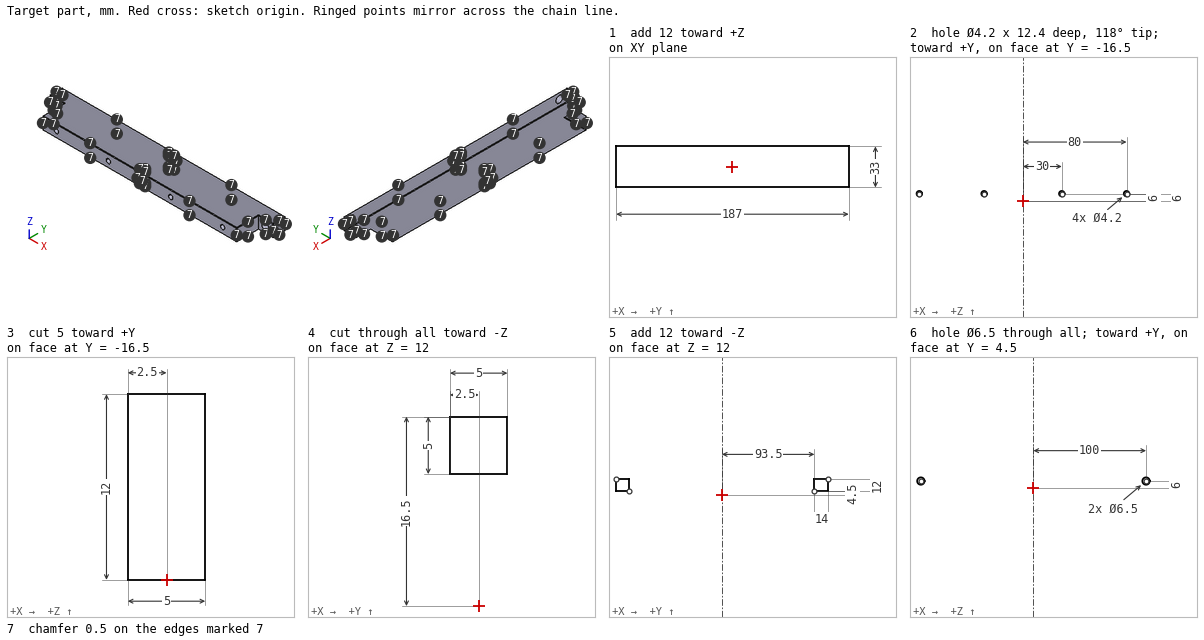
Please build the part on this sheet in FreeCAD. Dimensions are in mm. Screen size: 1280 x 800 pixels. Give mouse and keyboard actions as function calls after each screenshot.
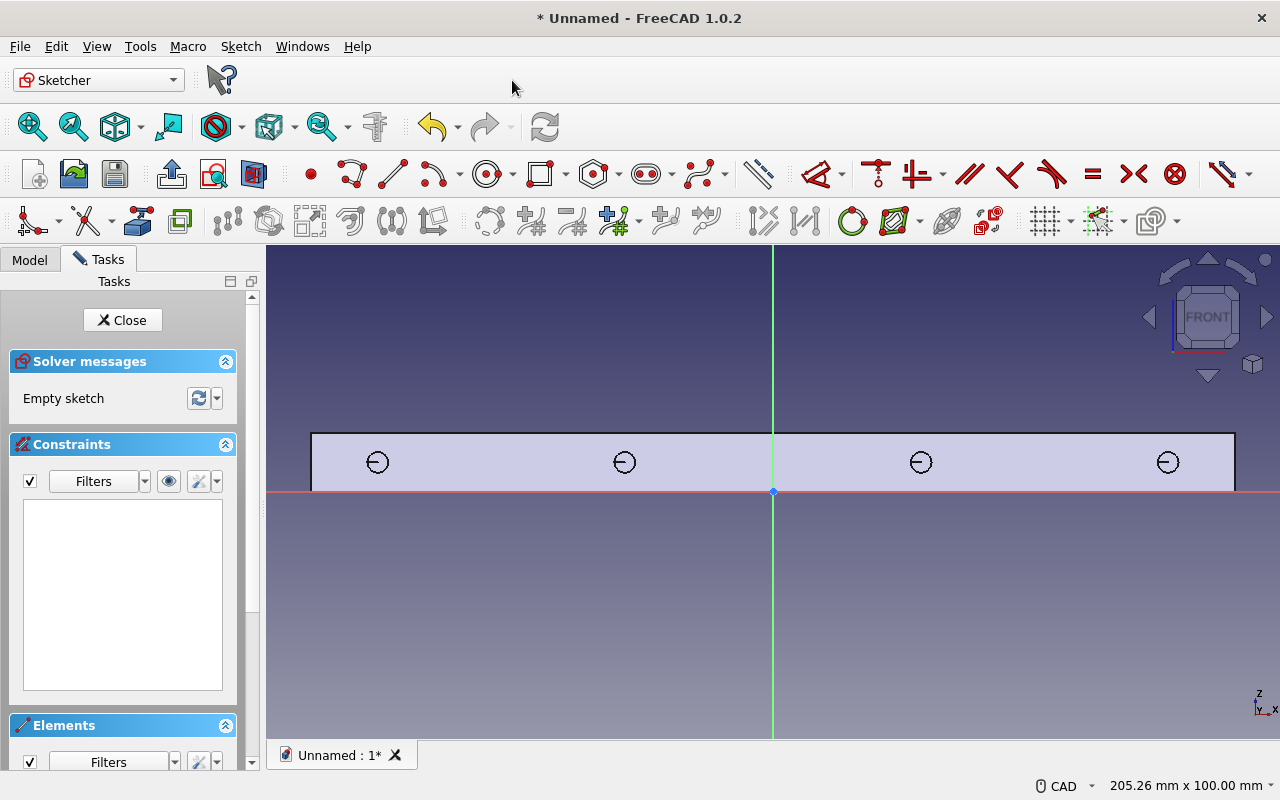
scroll(790, 455, up, 8)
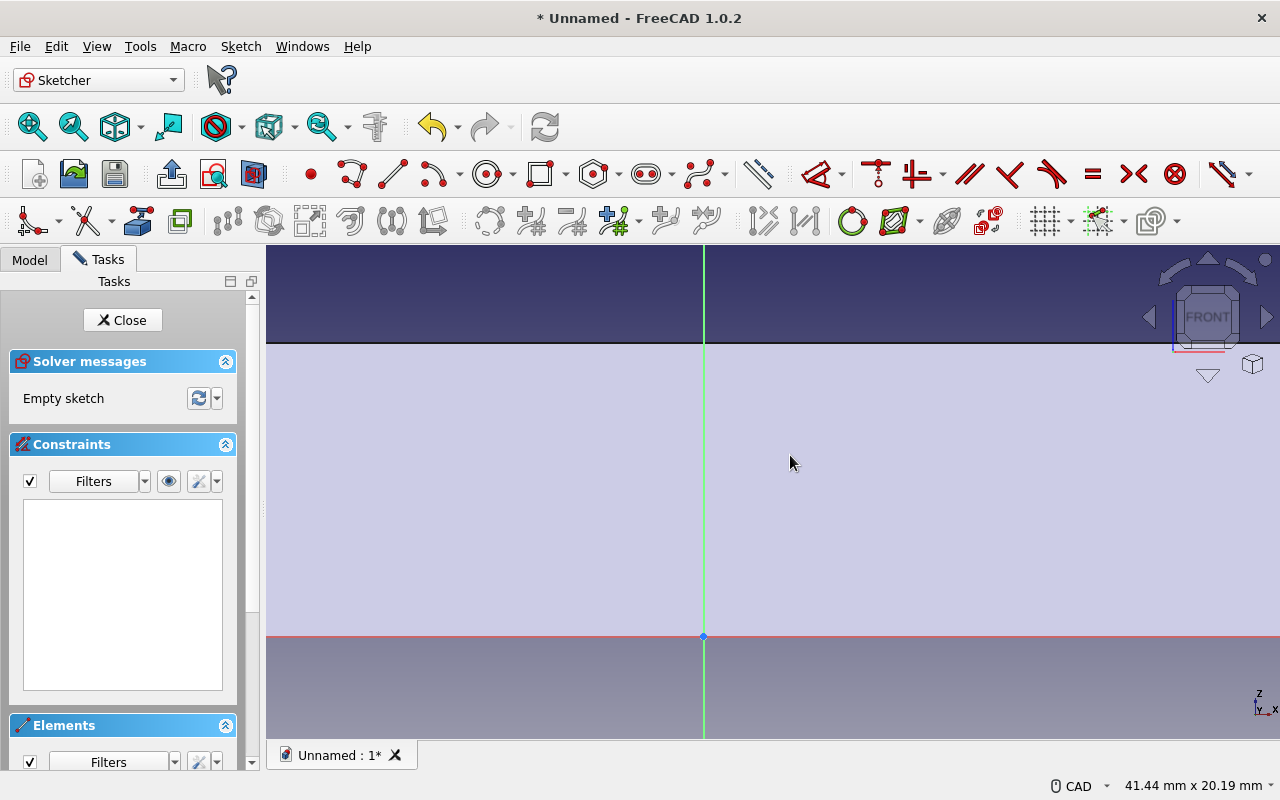
key(g)
key(r)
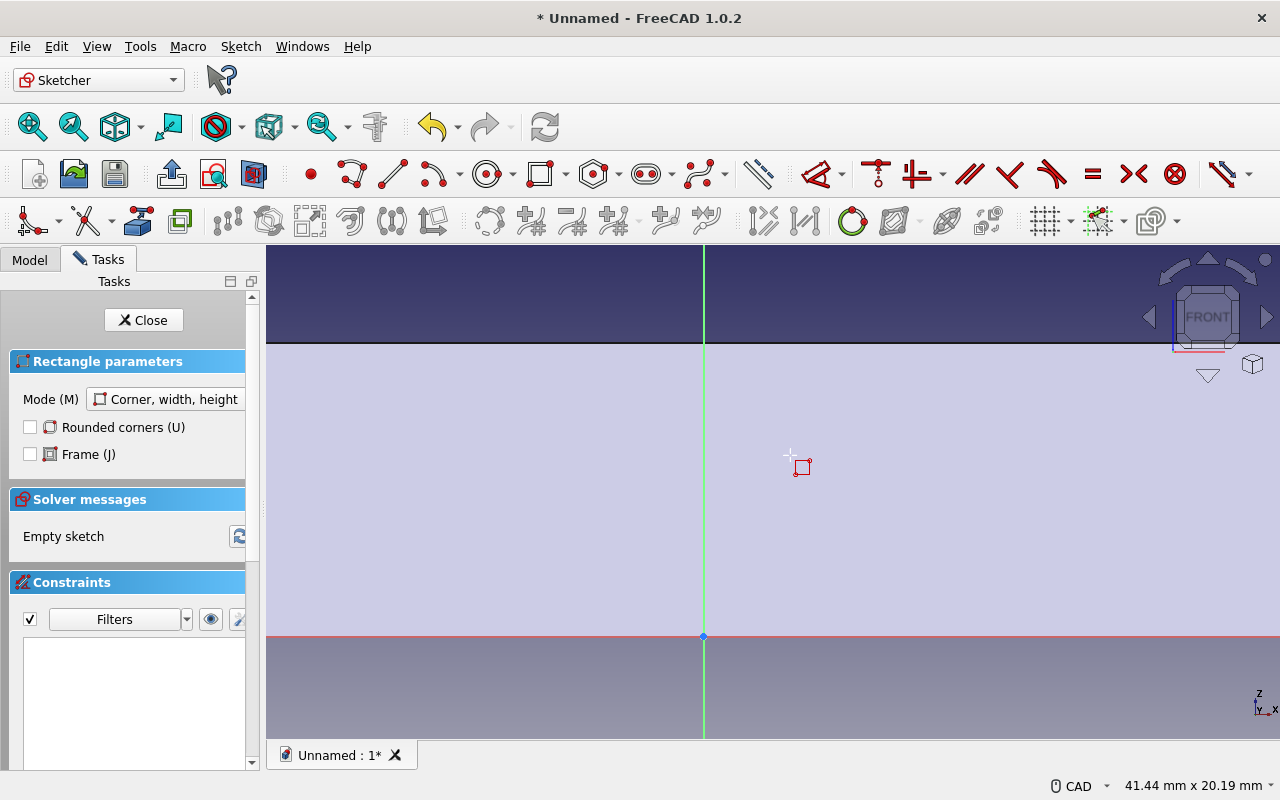
click(643, 343)
click(765, 637)
key(Escape)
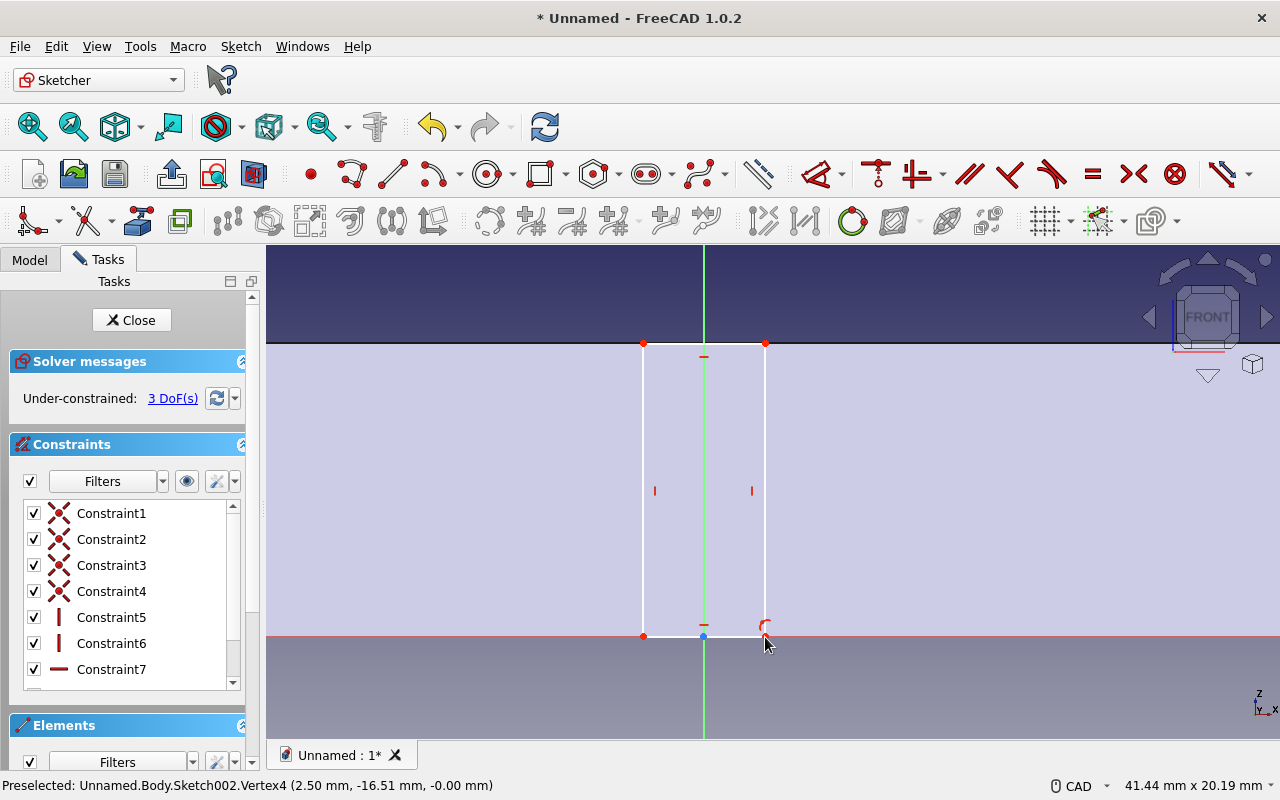
key(d)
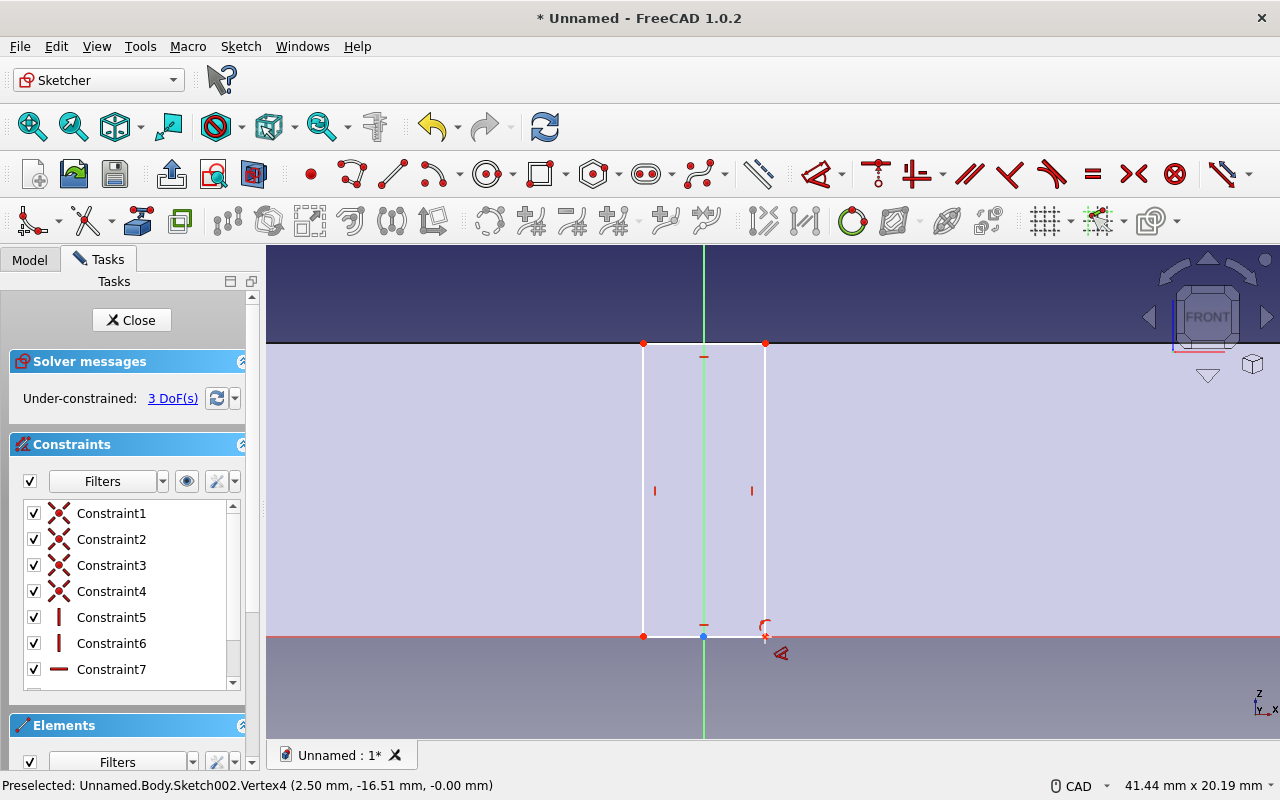
click(680, 637)
click(676, 671)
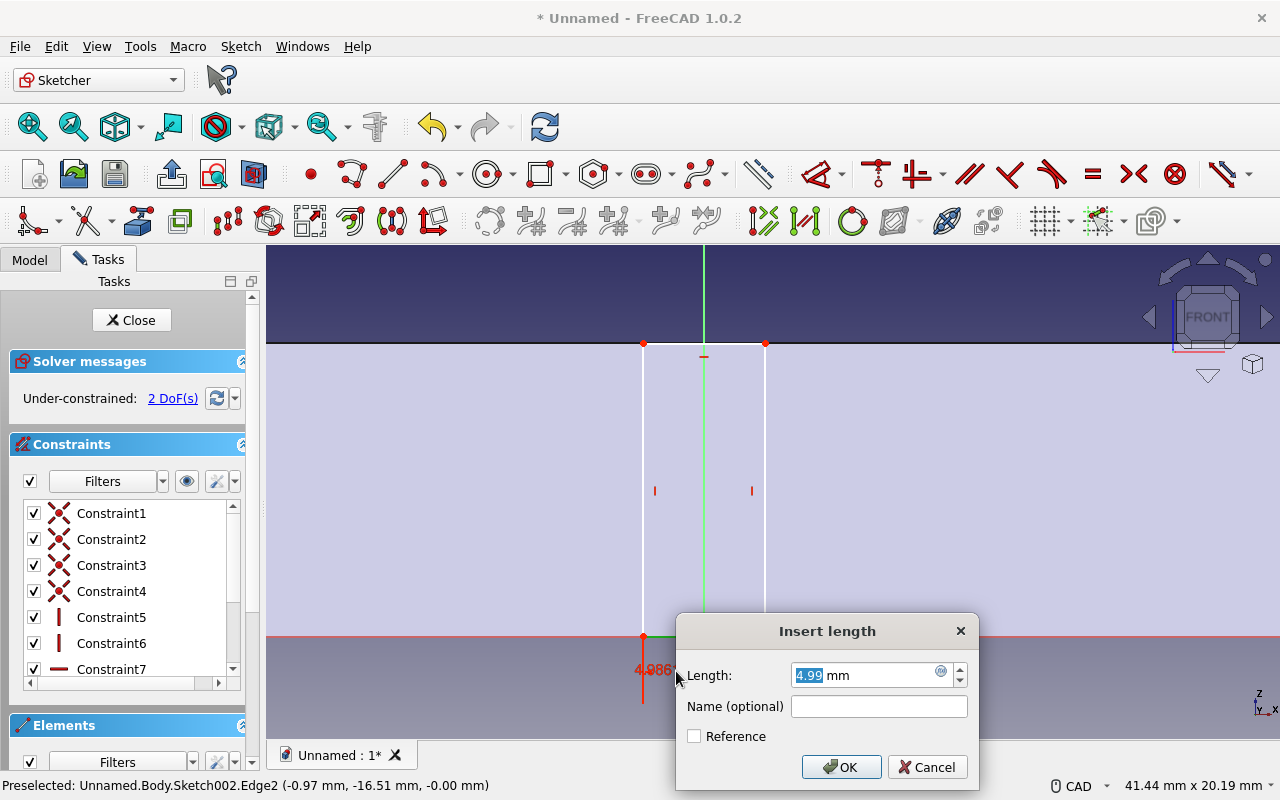
text(5)
key(Return)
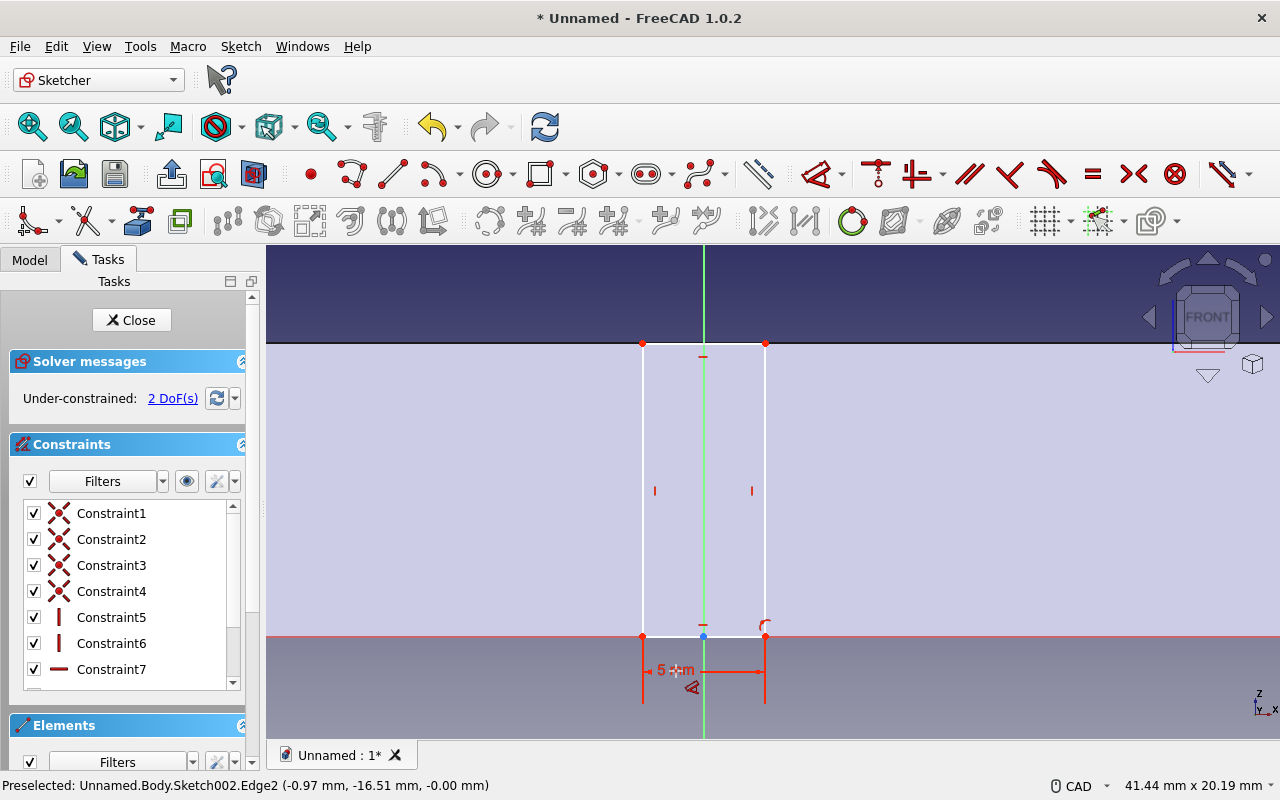
click(643, 432)
click(609, 490)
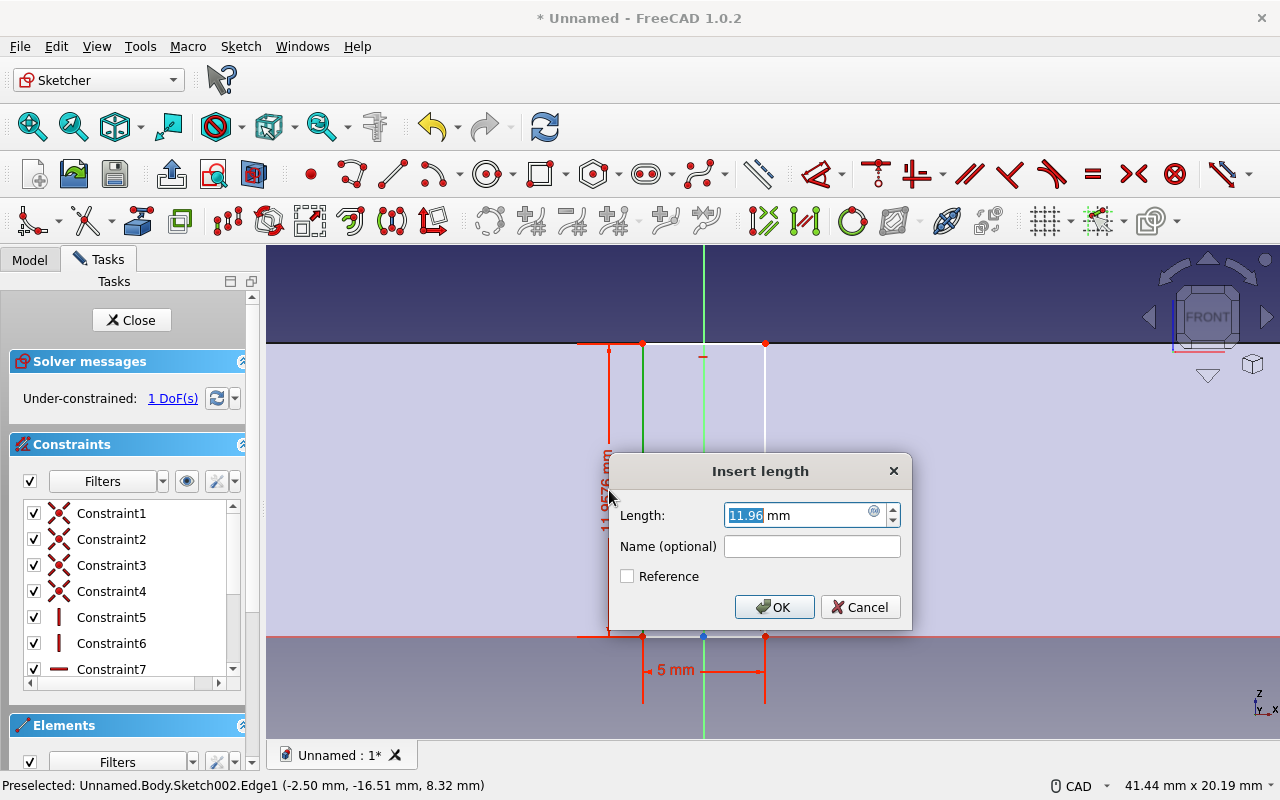
text(12)
key(Return)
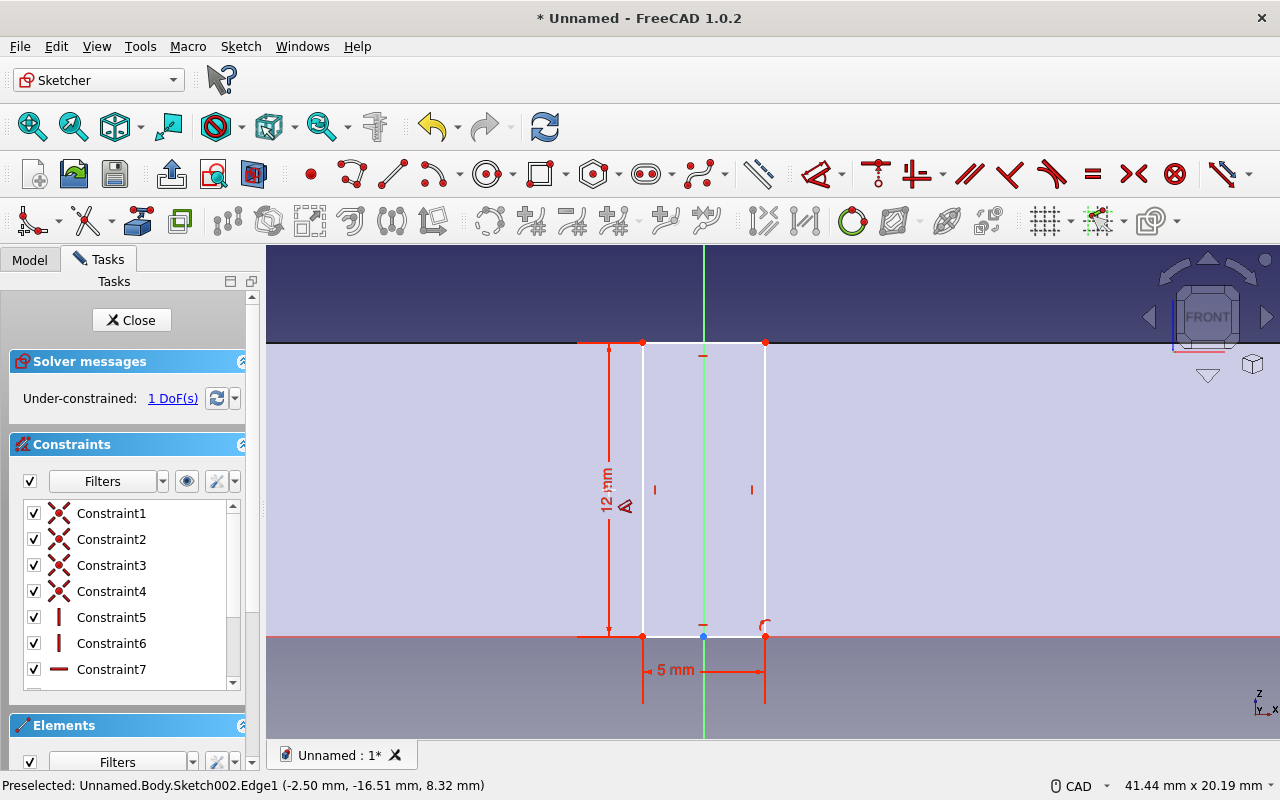
click(643, 343)
click(673, 309)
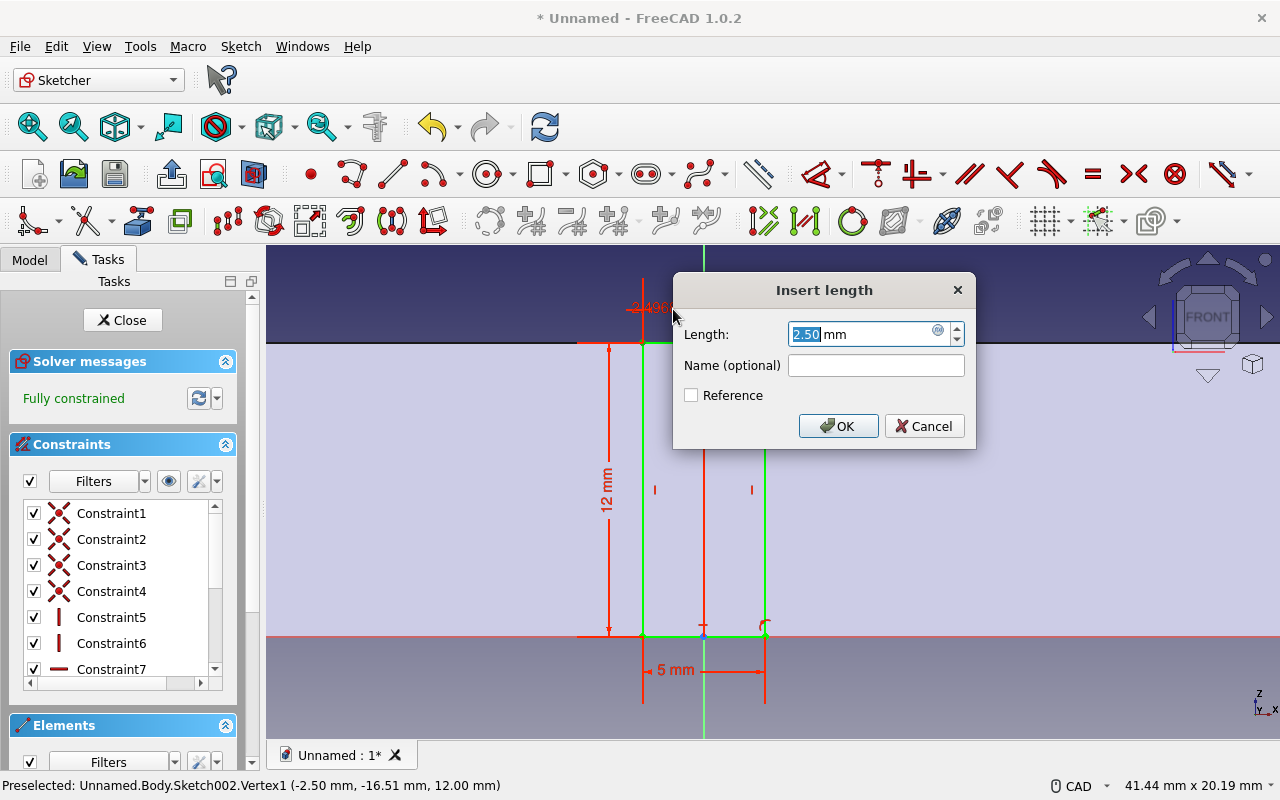
text(2.5)
key(Return)
key(Escape)